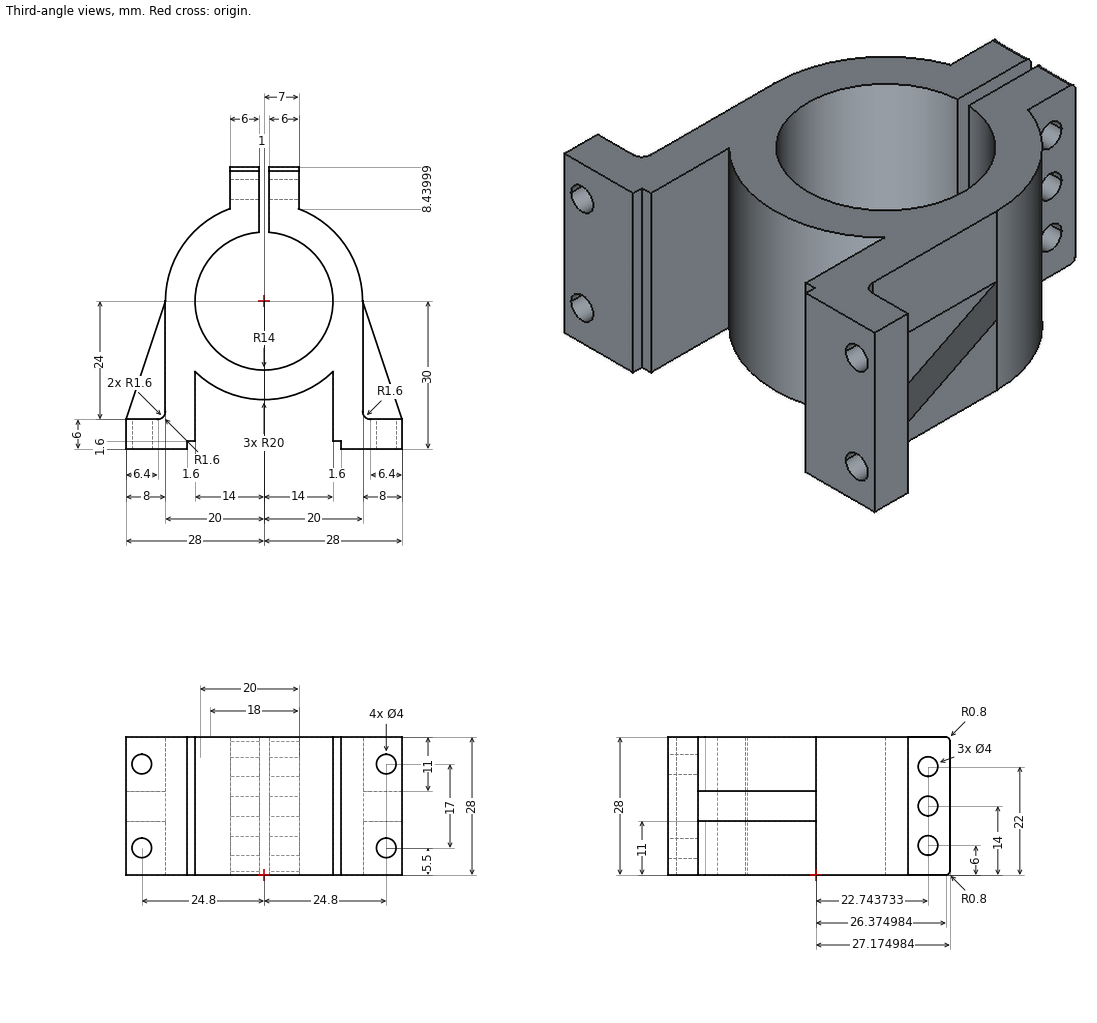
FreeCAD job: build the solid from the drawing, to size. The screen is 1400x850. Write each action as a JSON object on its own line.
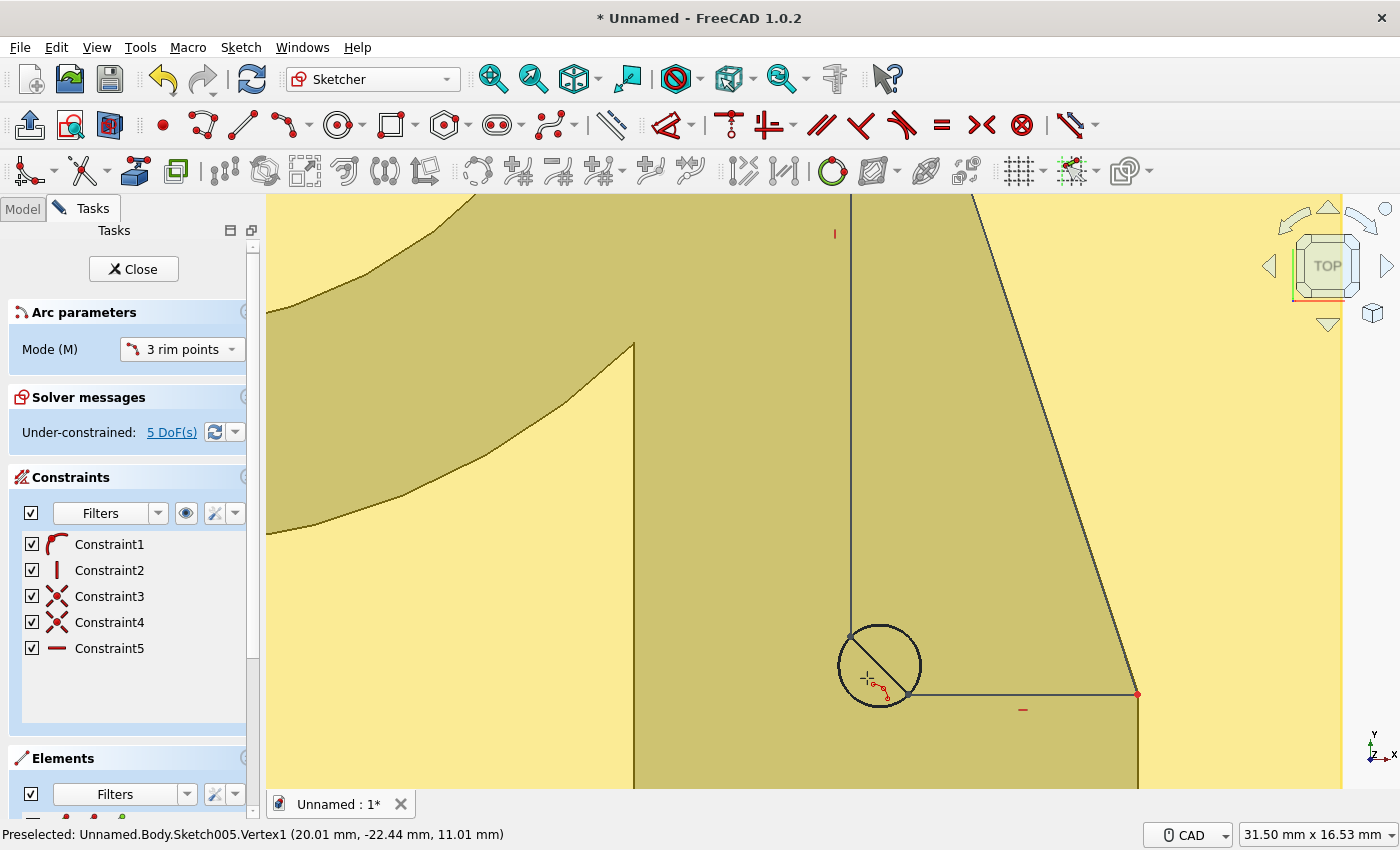
{"action": "left_click", "coordinate": [867, 676]}
{"action": "key", "text": "Escape"}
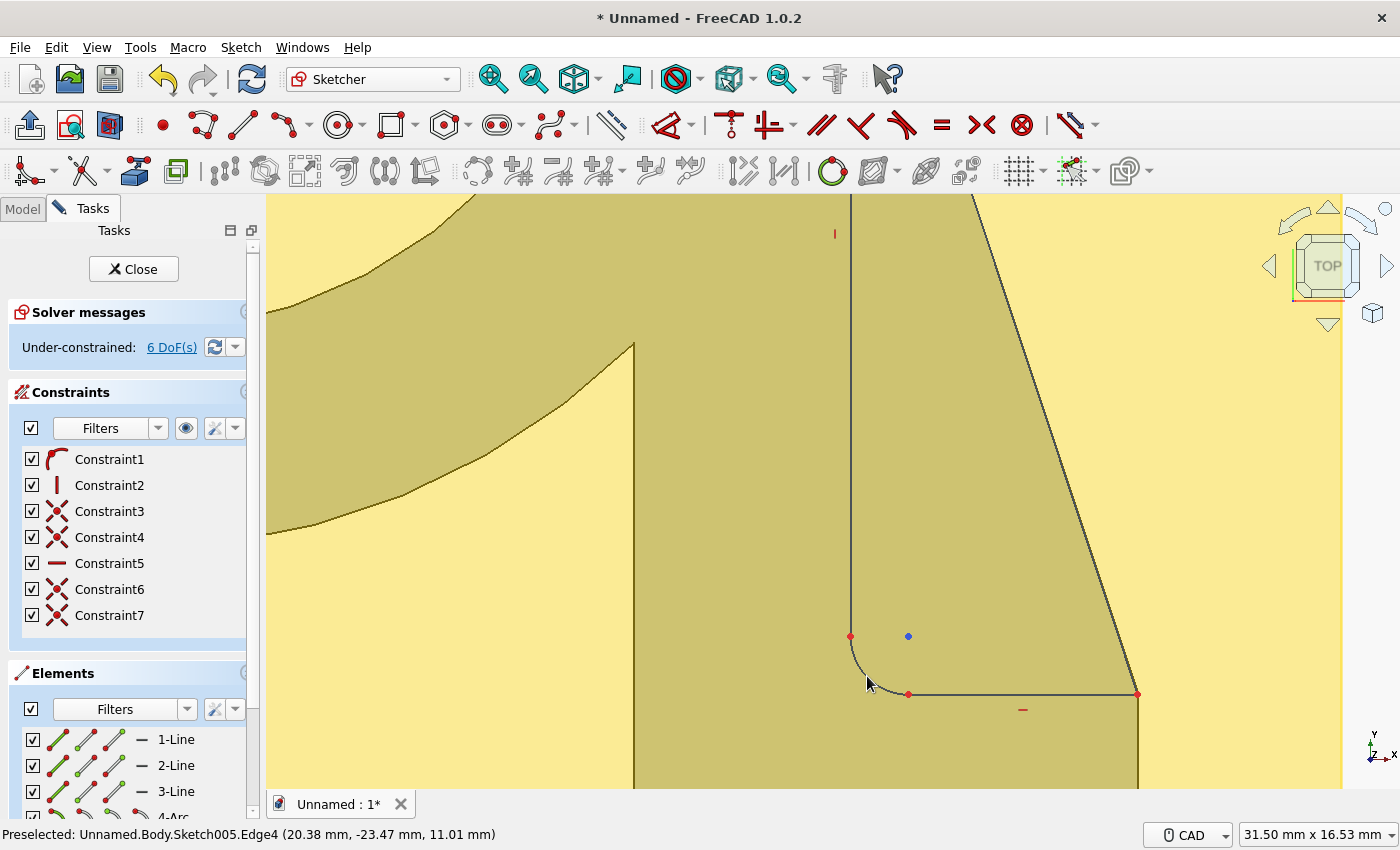
{"action": "left_click", "coordinate": [851, 395]}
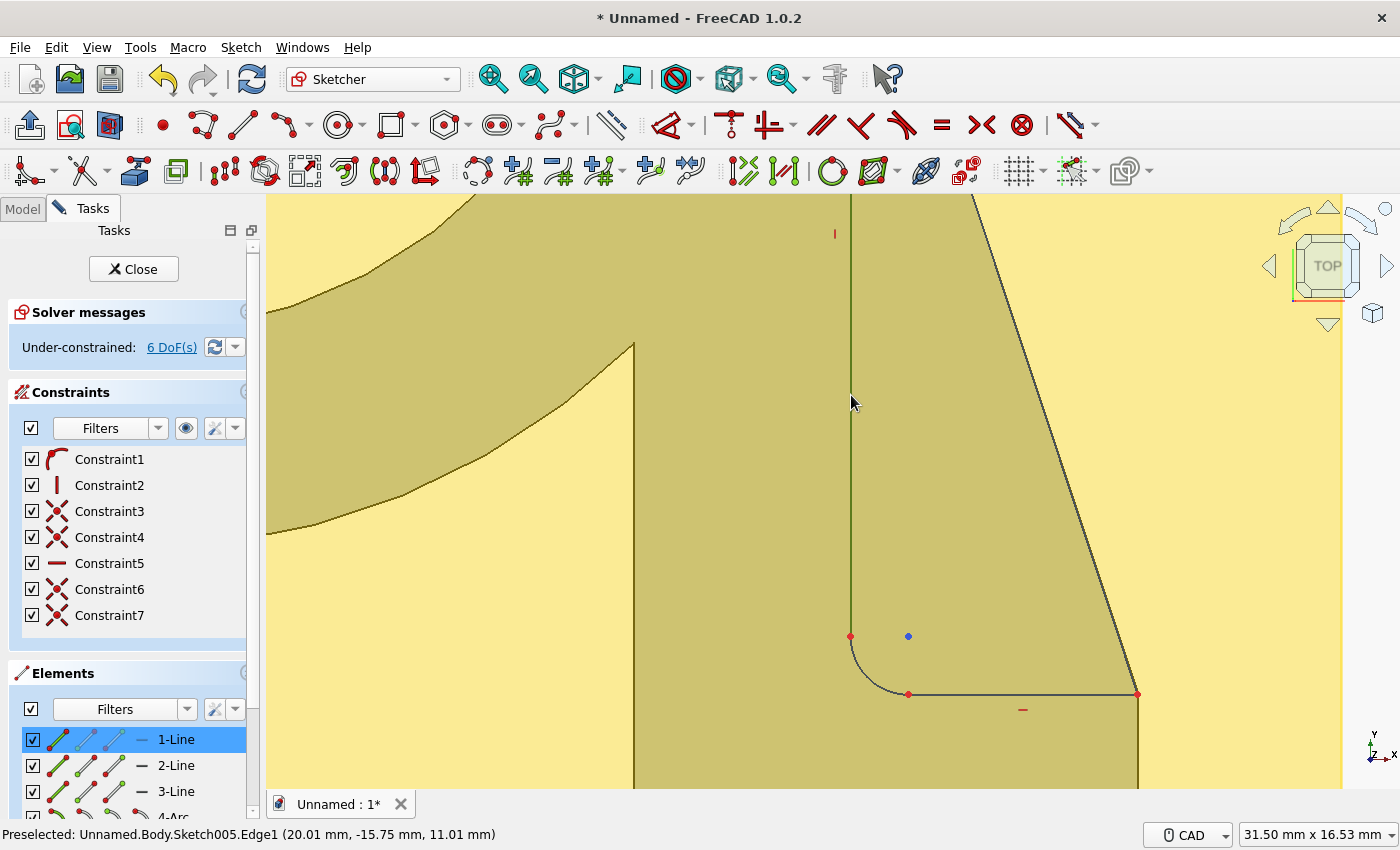
{"action": "left_click", "coordinate": [857, 663]}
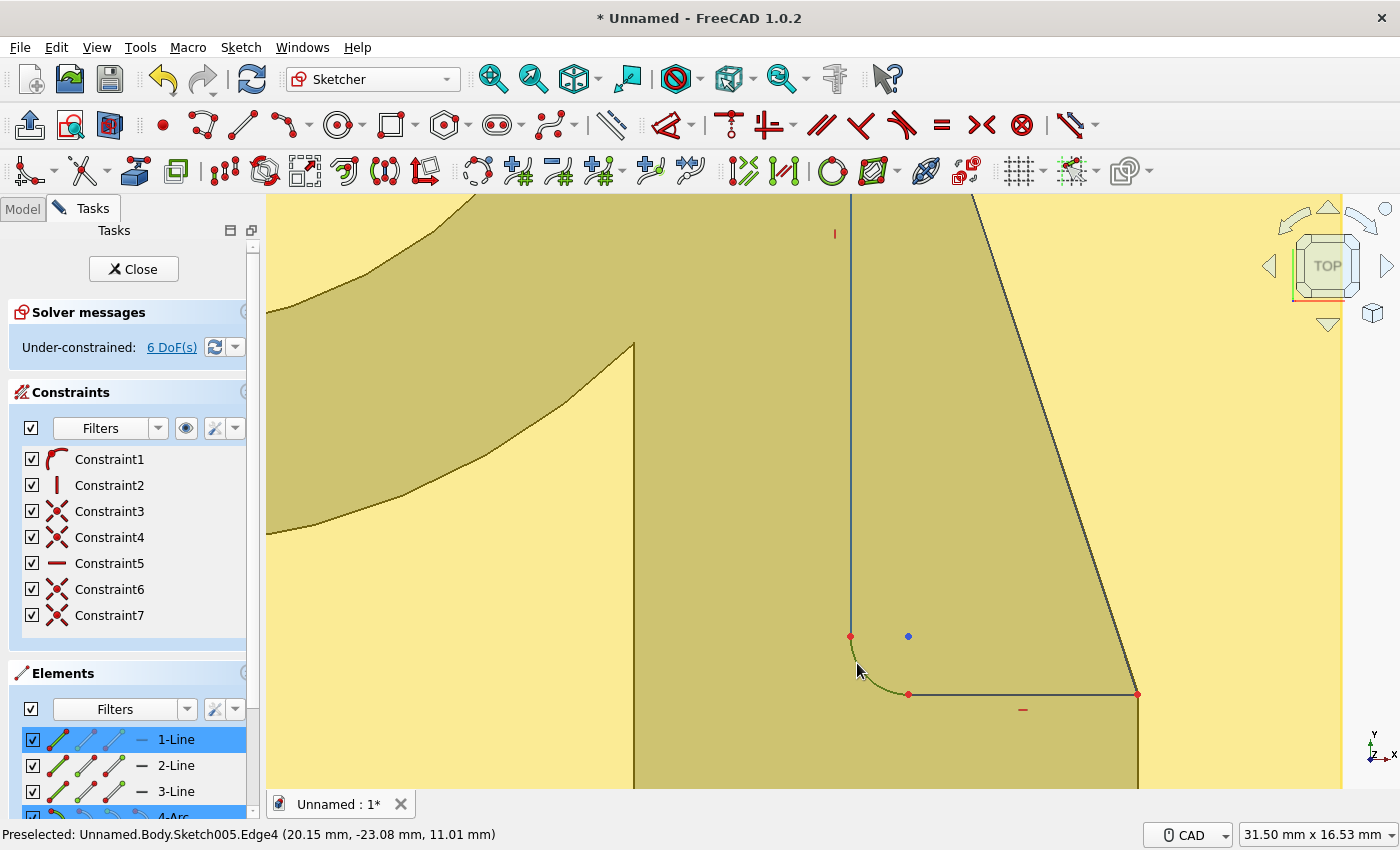
{"action": "left_click", "coordinate": [902, 126]}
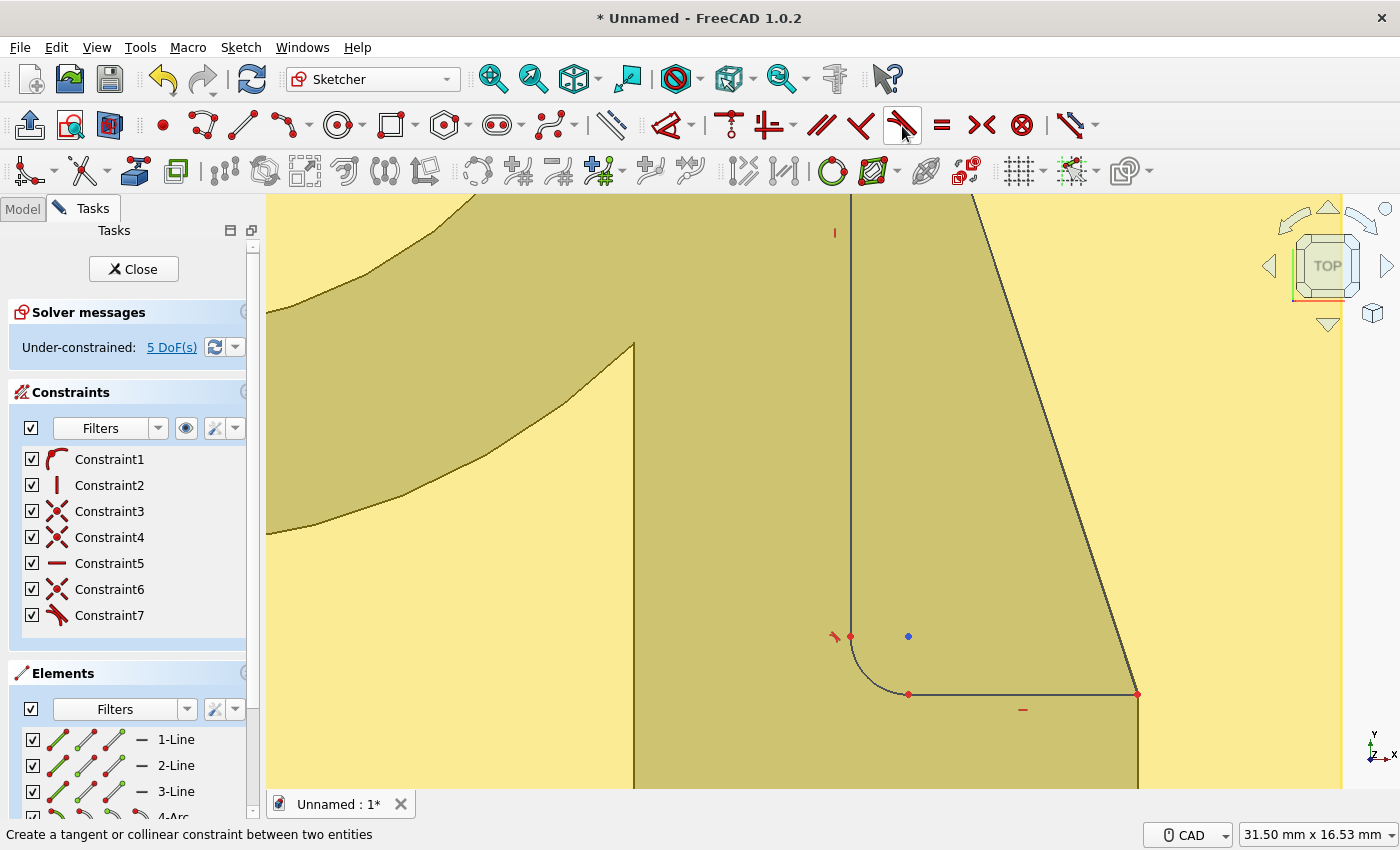
{"action": "left_click", "coordinate": [1069, 695]}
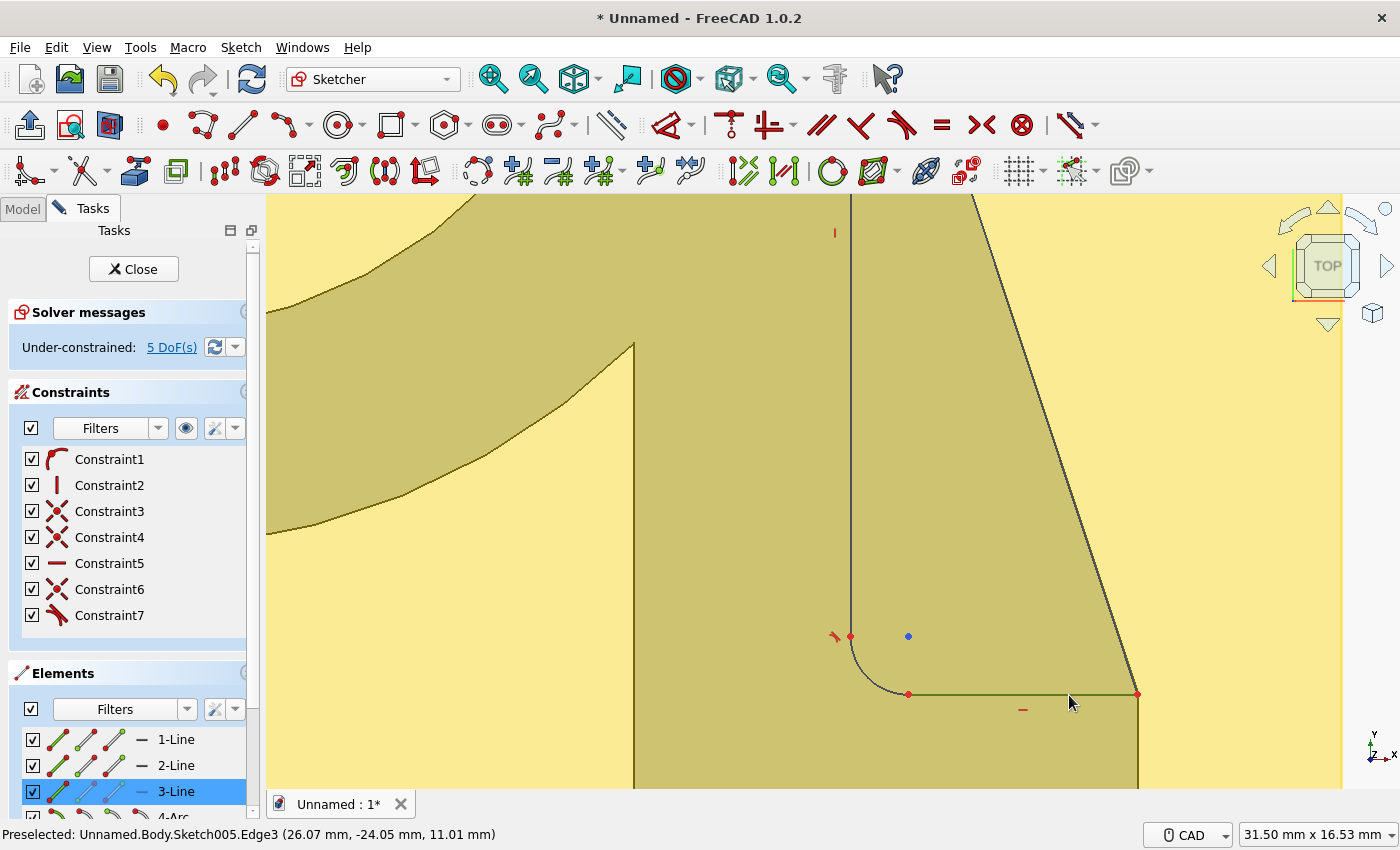
{"action": "left_click", "coordinate": [857, 663]}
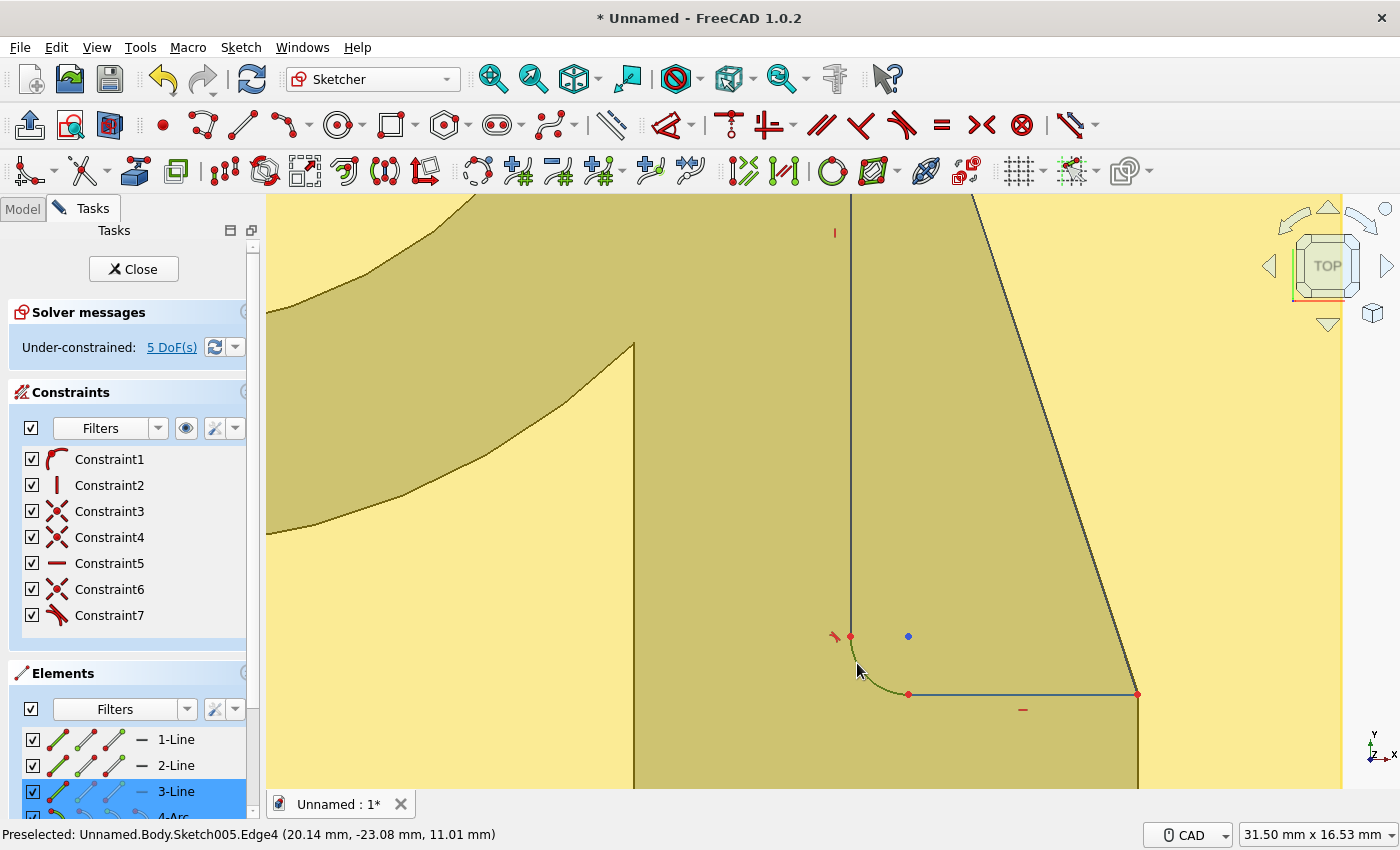
{"action": "left_click", "coordinate": [902, 126]}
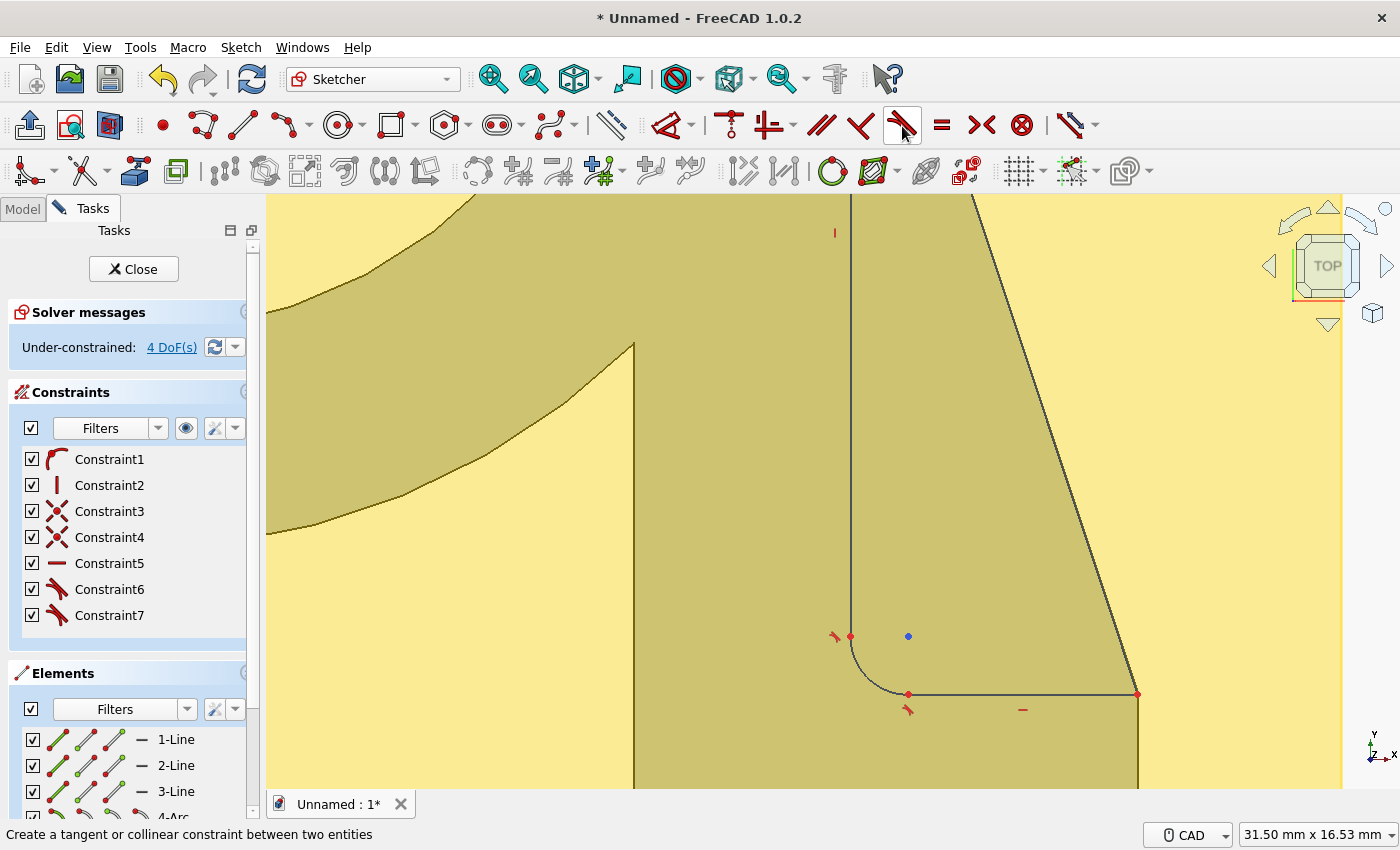
{"action": "left_click", "coordinate": [666, 126]}